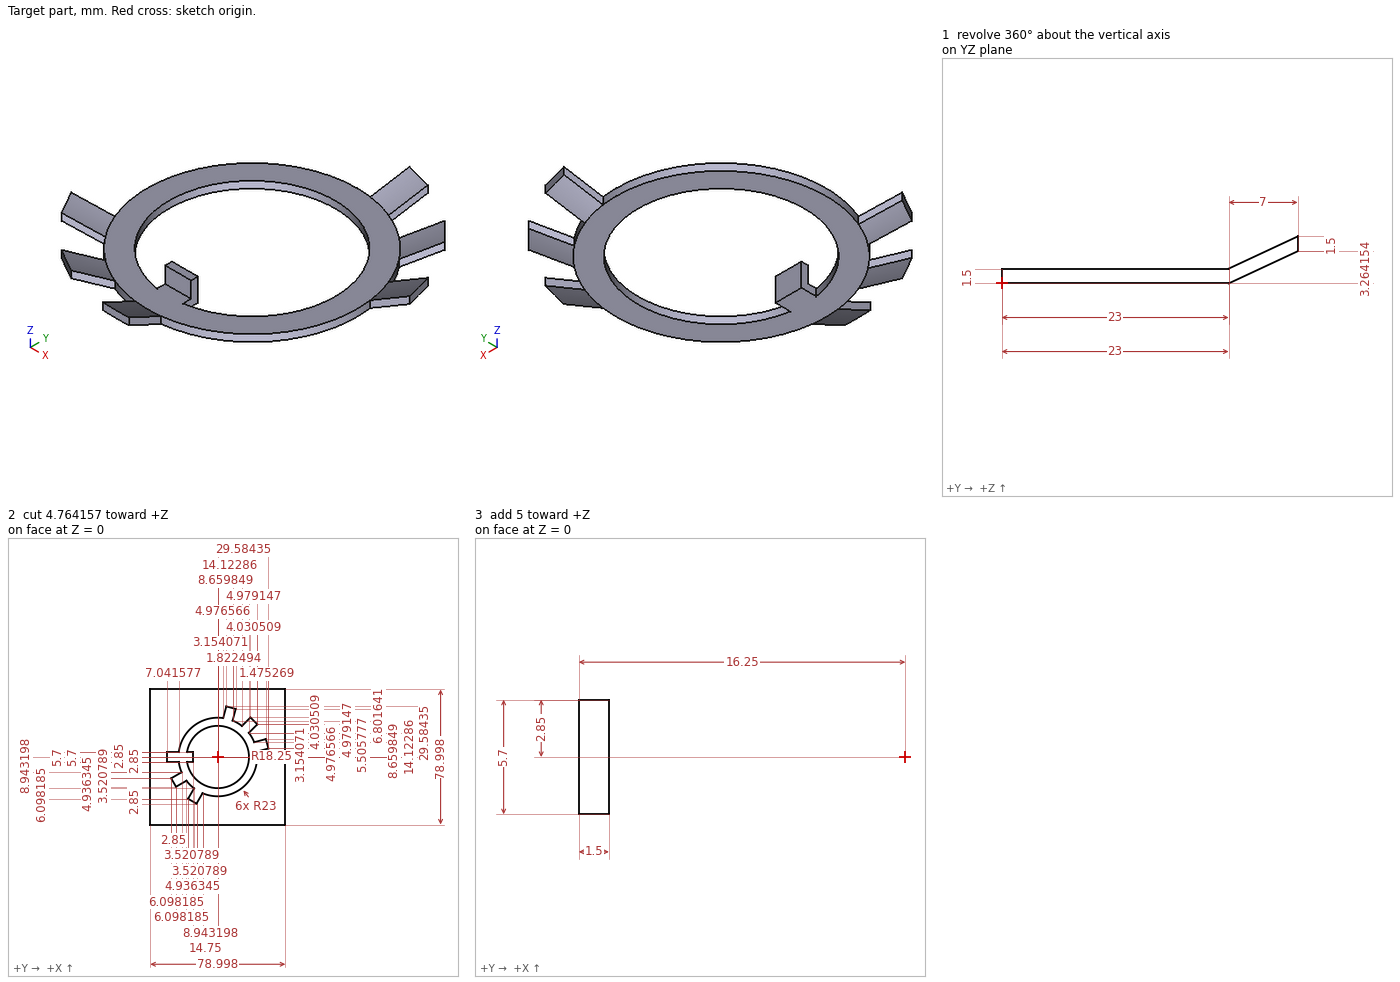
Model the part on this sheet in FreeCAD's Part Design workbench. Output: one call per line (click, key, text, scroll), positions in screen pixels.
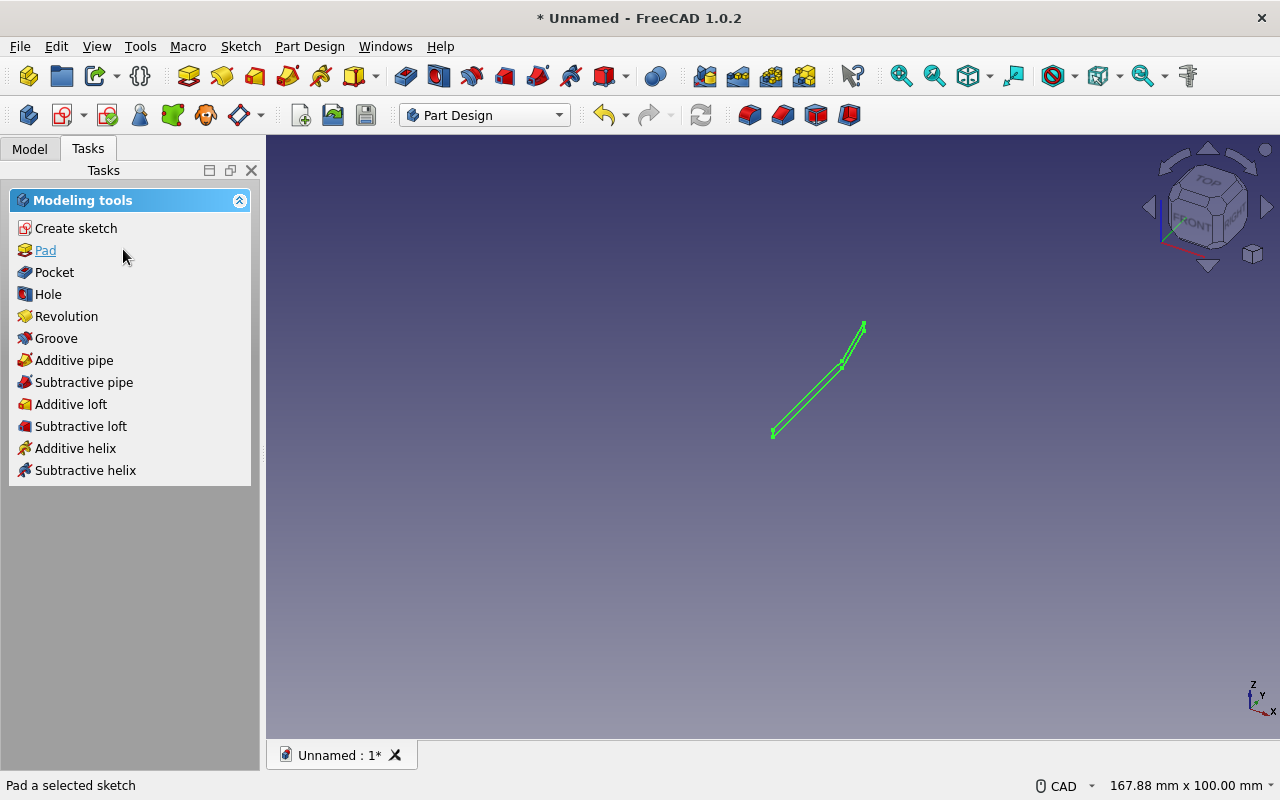
click(222, 76)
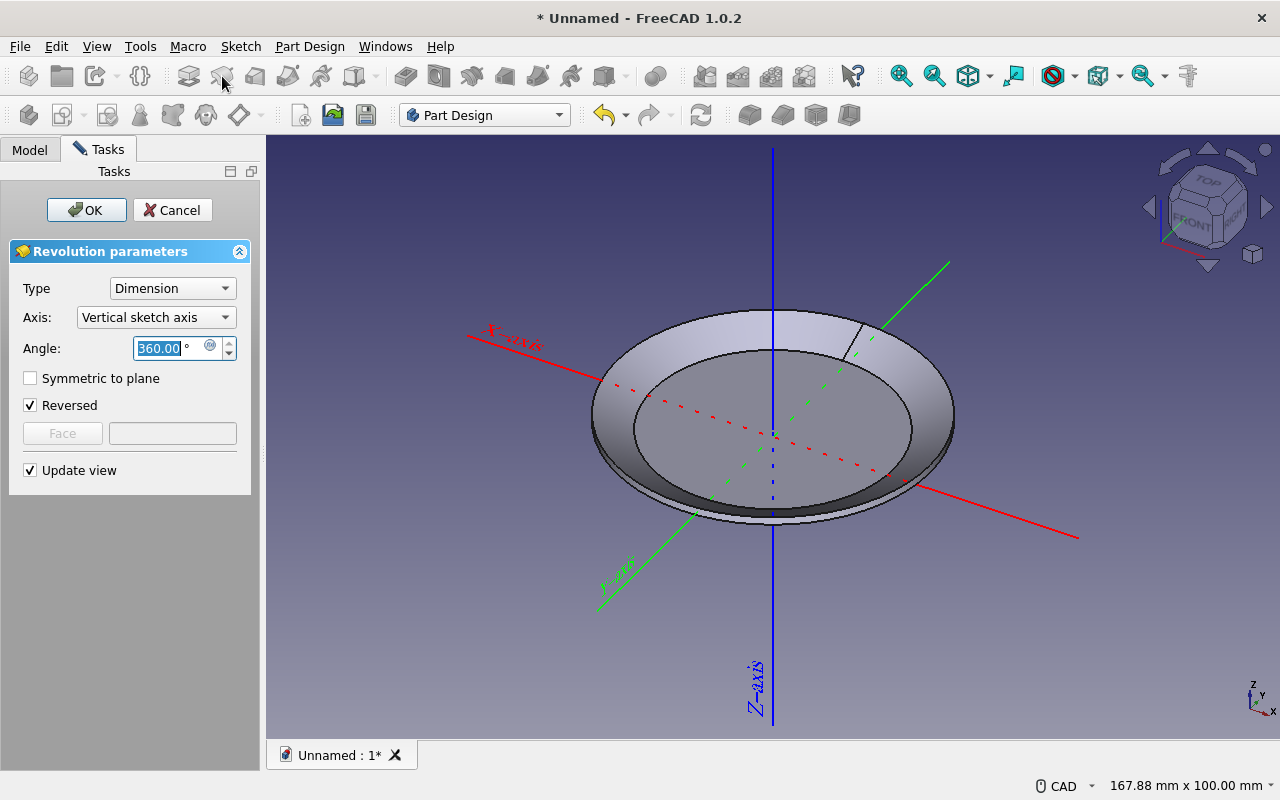
click(87, 210)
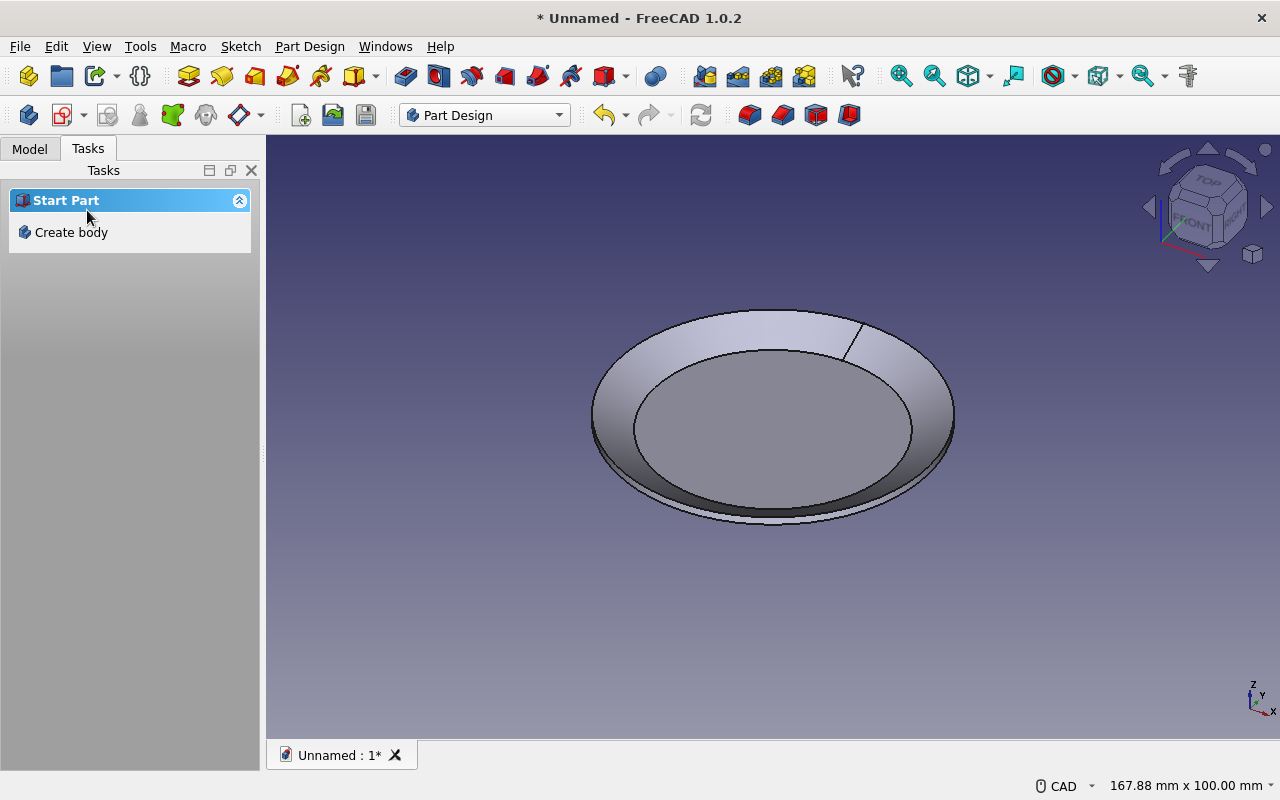
key(5)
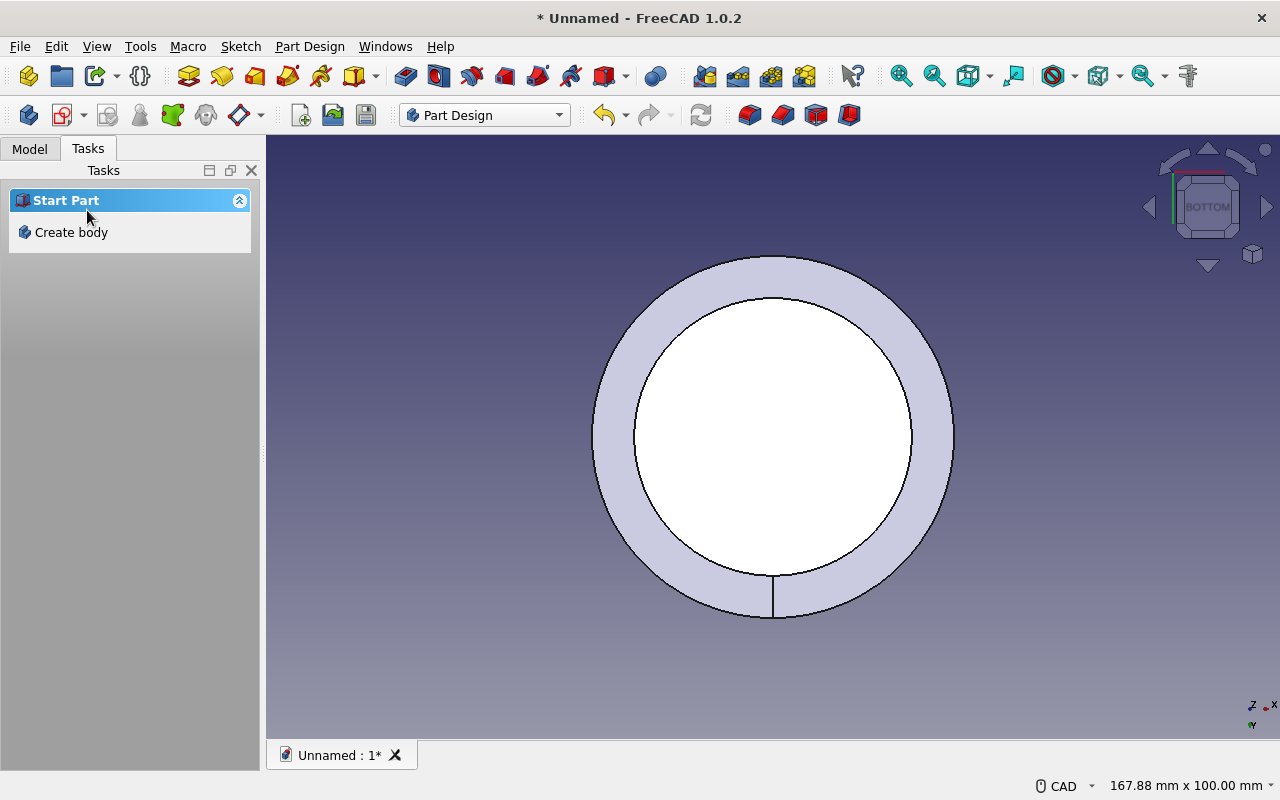
click(773, 436)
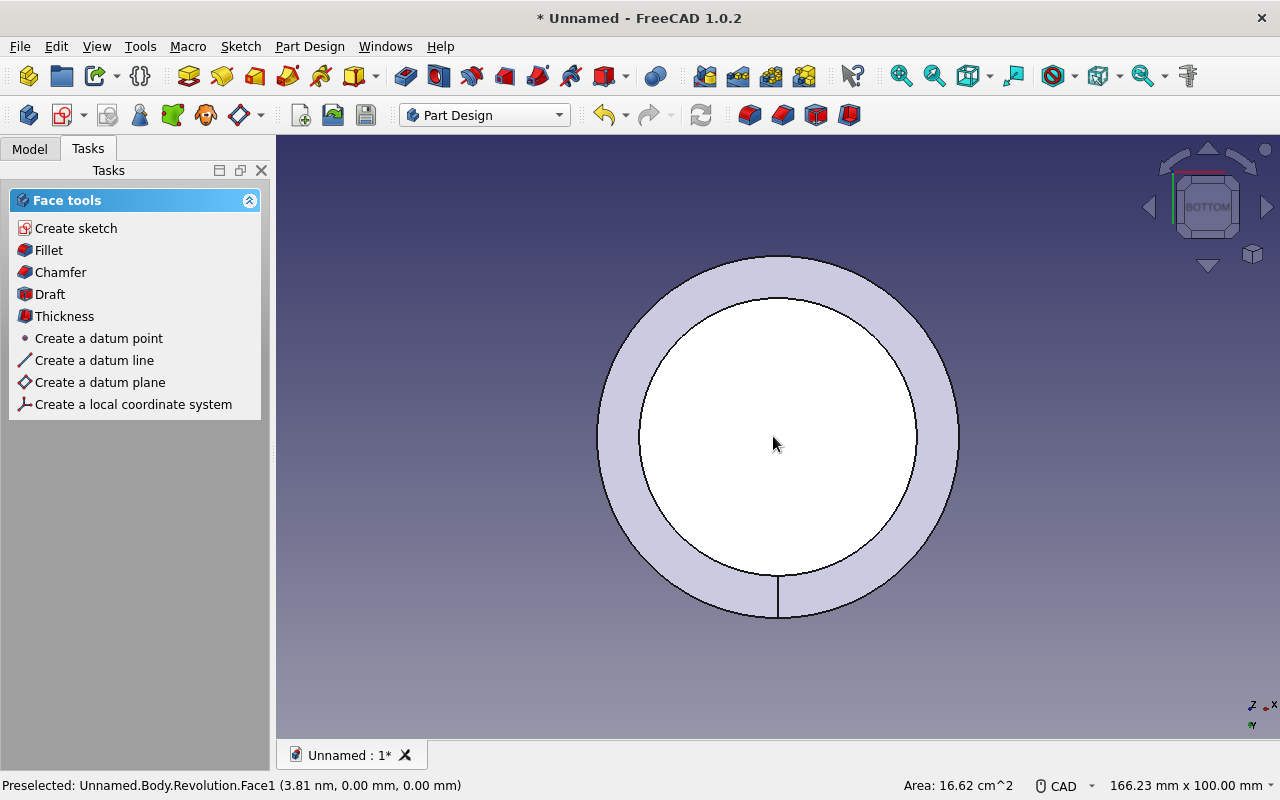
click(62, 116)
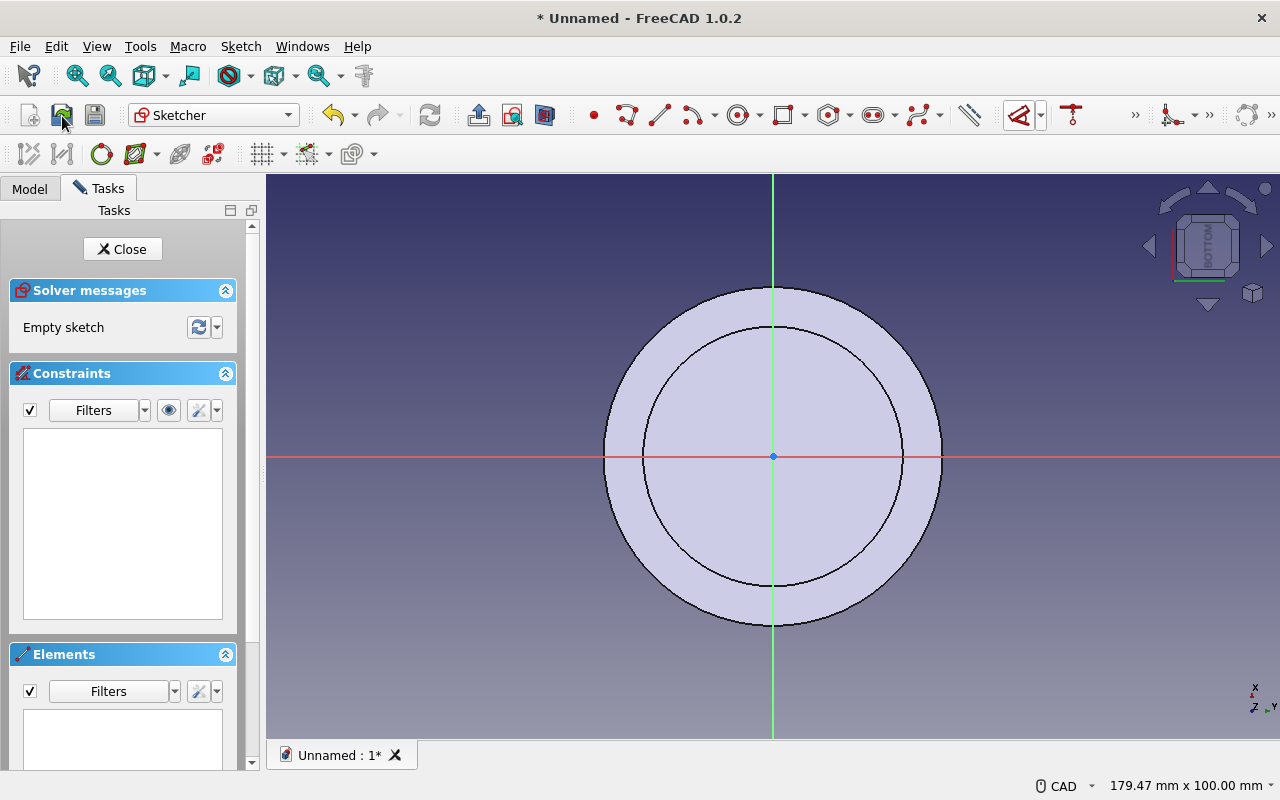
key(g)
key(v)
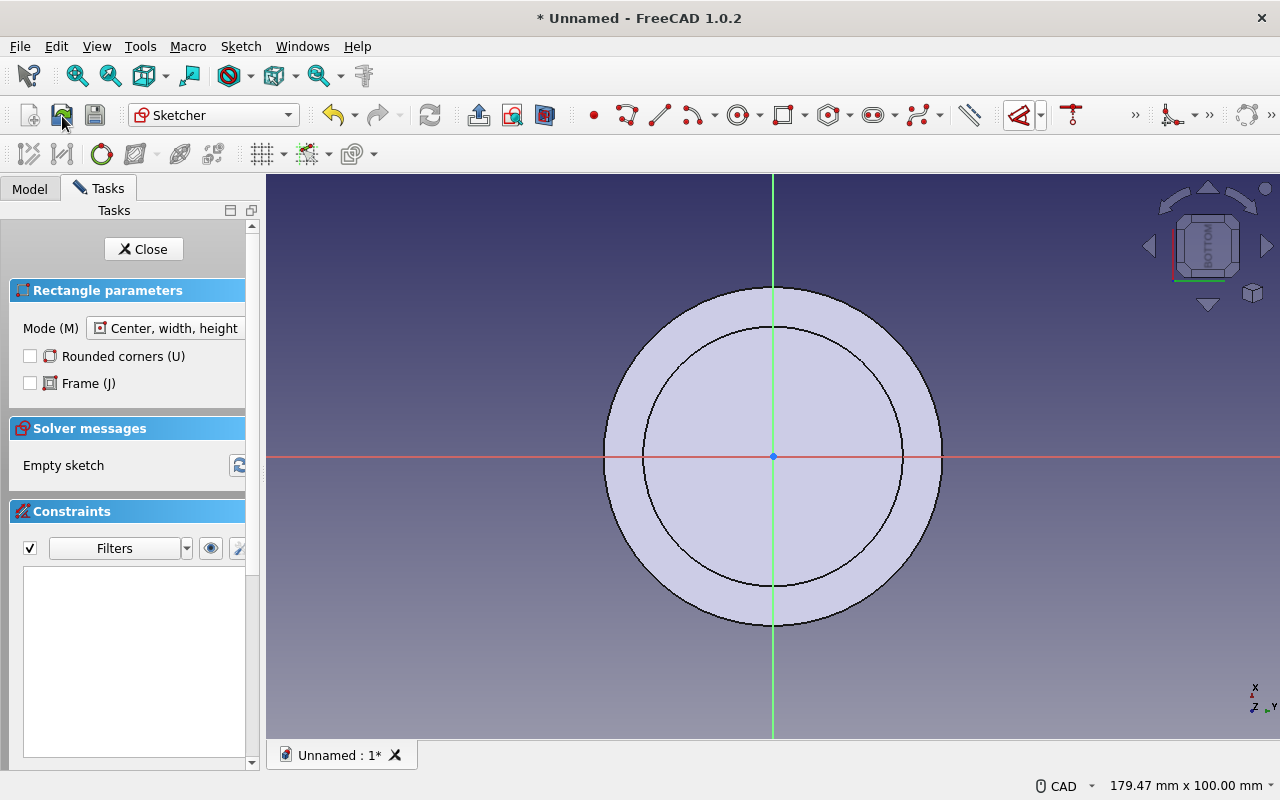
click(773, 457)
move(996, 233)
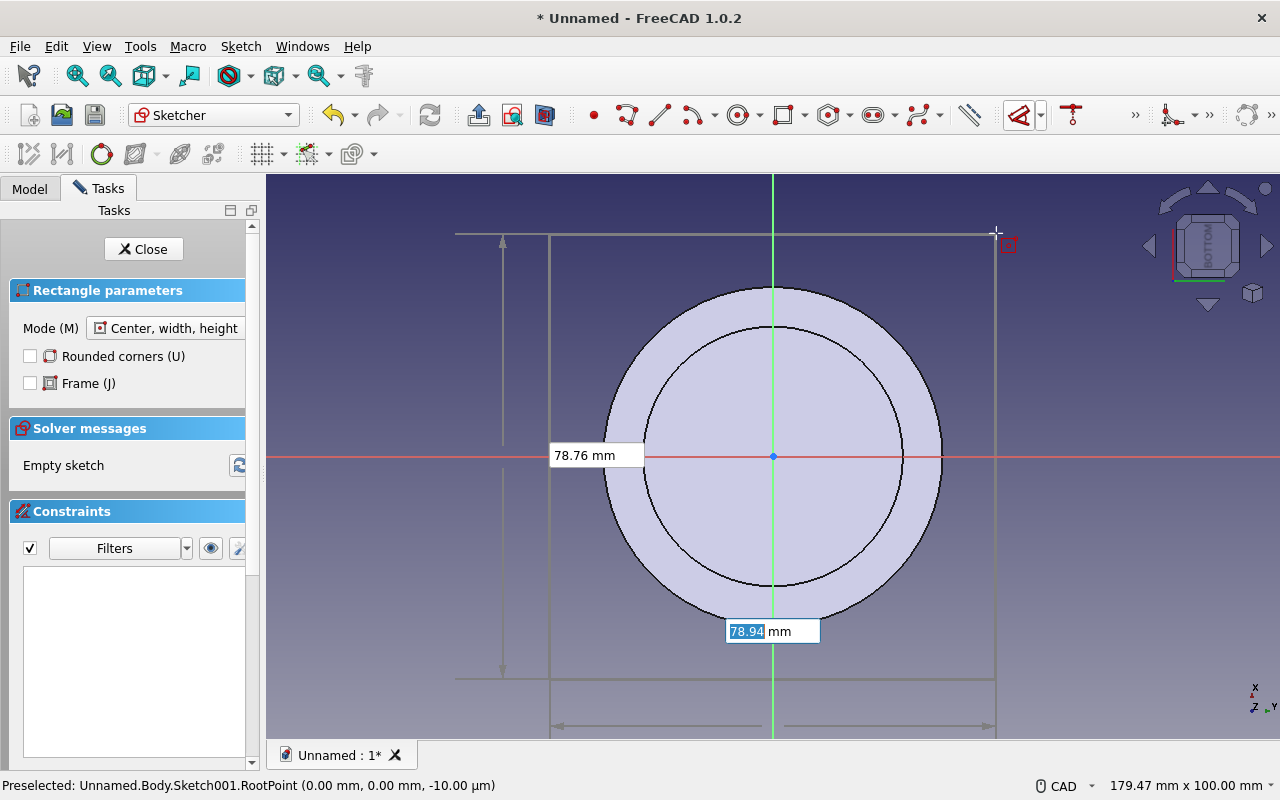
text(78.998)
key(Tab)
text(78.998)
key(Return)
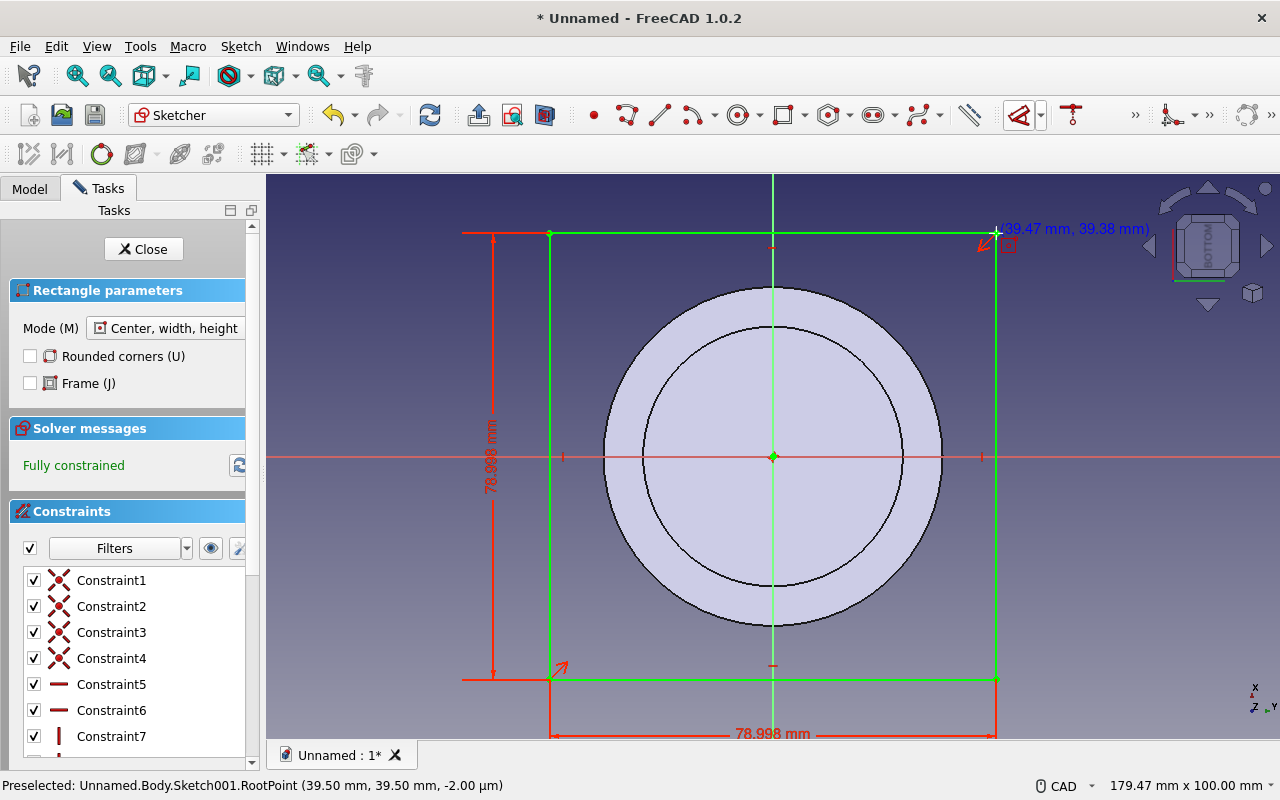
click(627, 116)